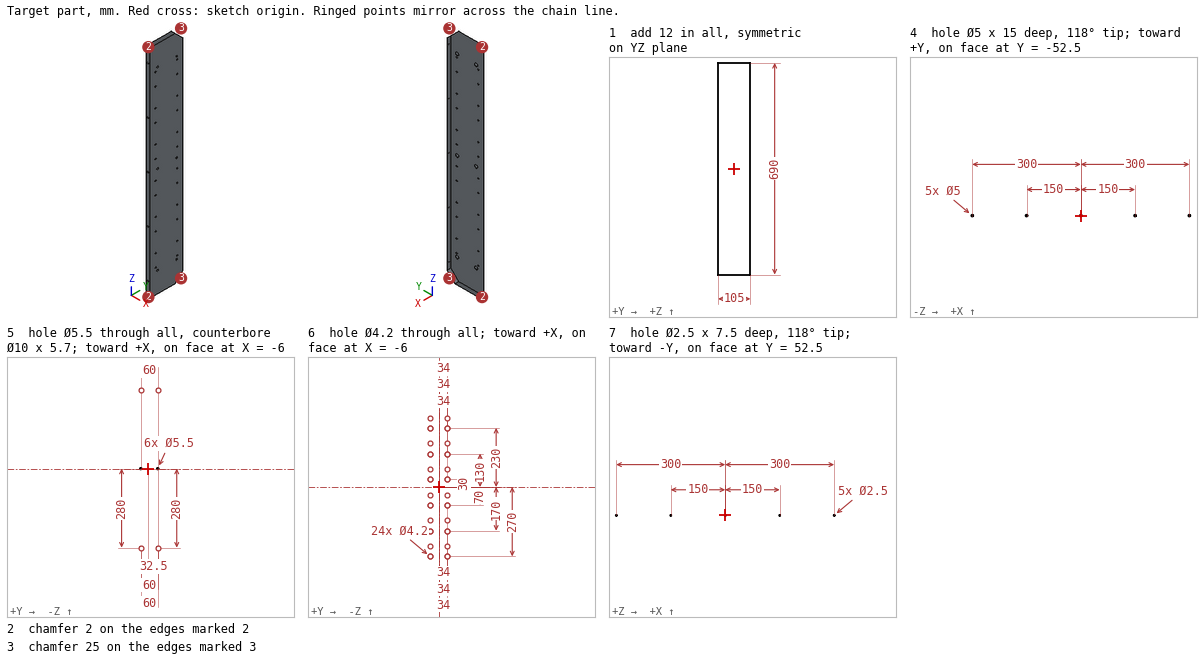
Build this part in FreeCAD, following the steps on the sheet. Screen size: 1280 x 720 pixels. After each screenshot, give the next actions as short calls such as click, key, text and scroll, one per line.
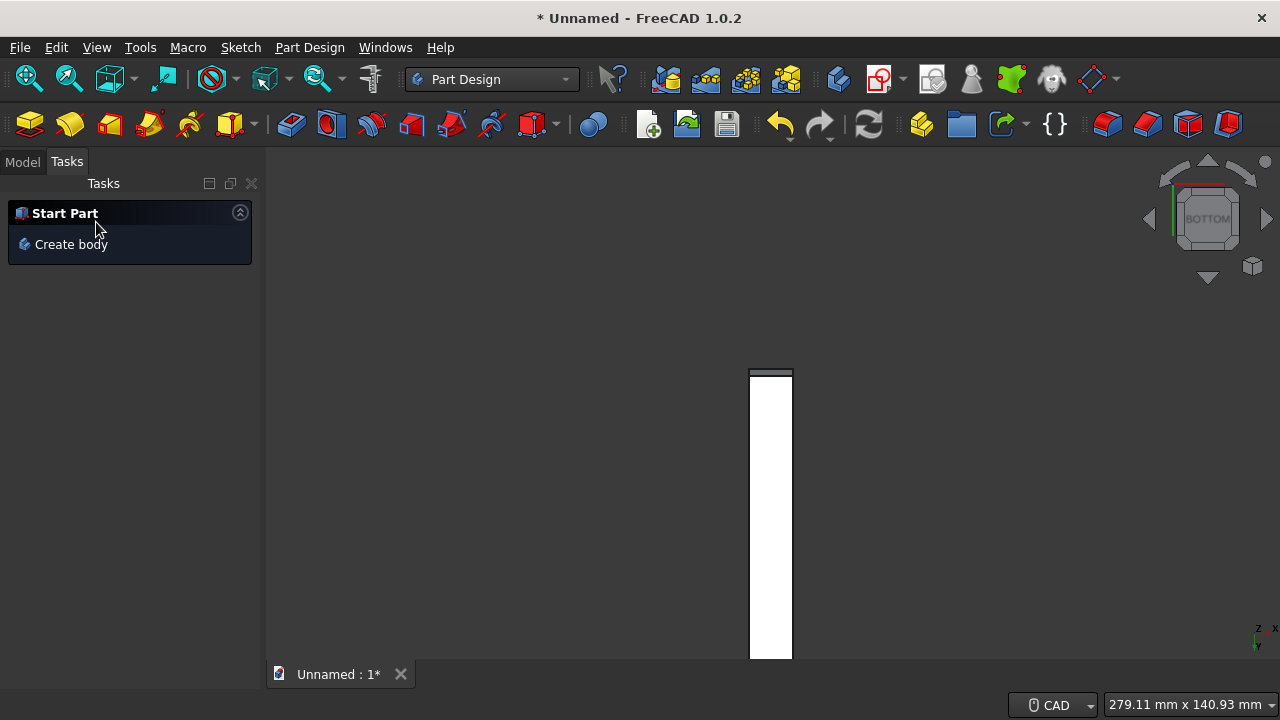
click(30, 80)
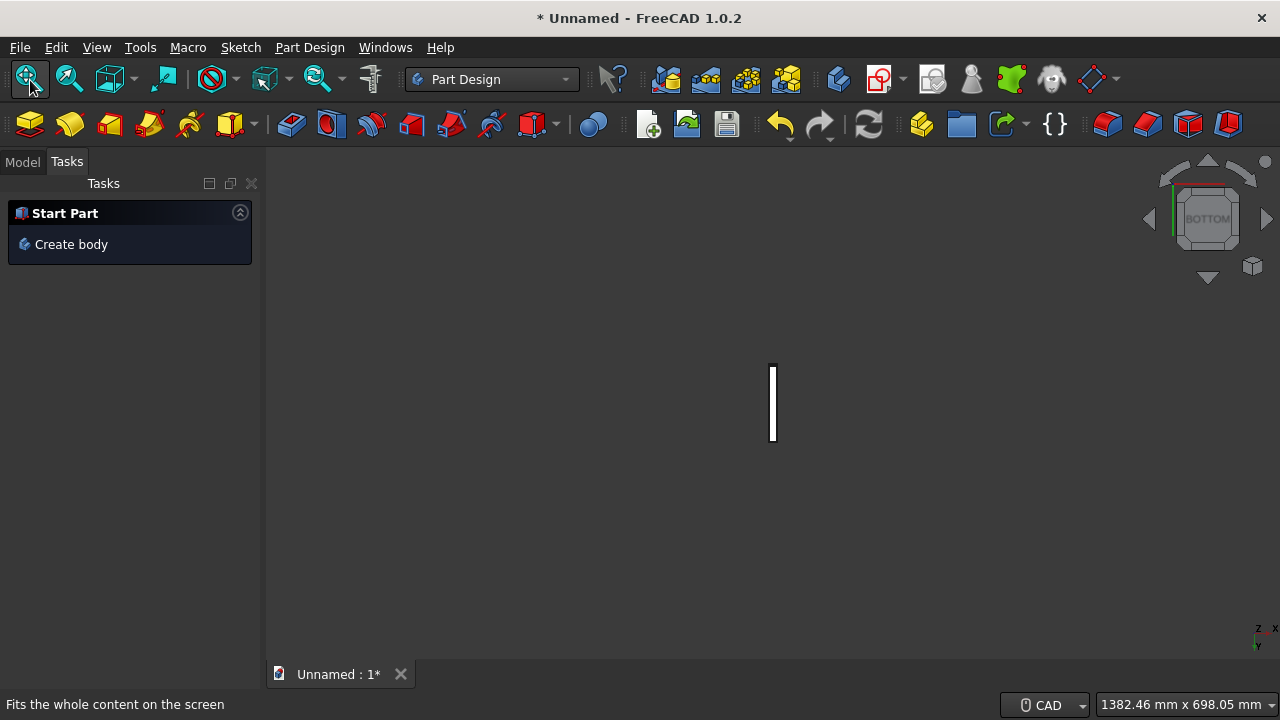
scroll(773, 441, up, 8)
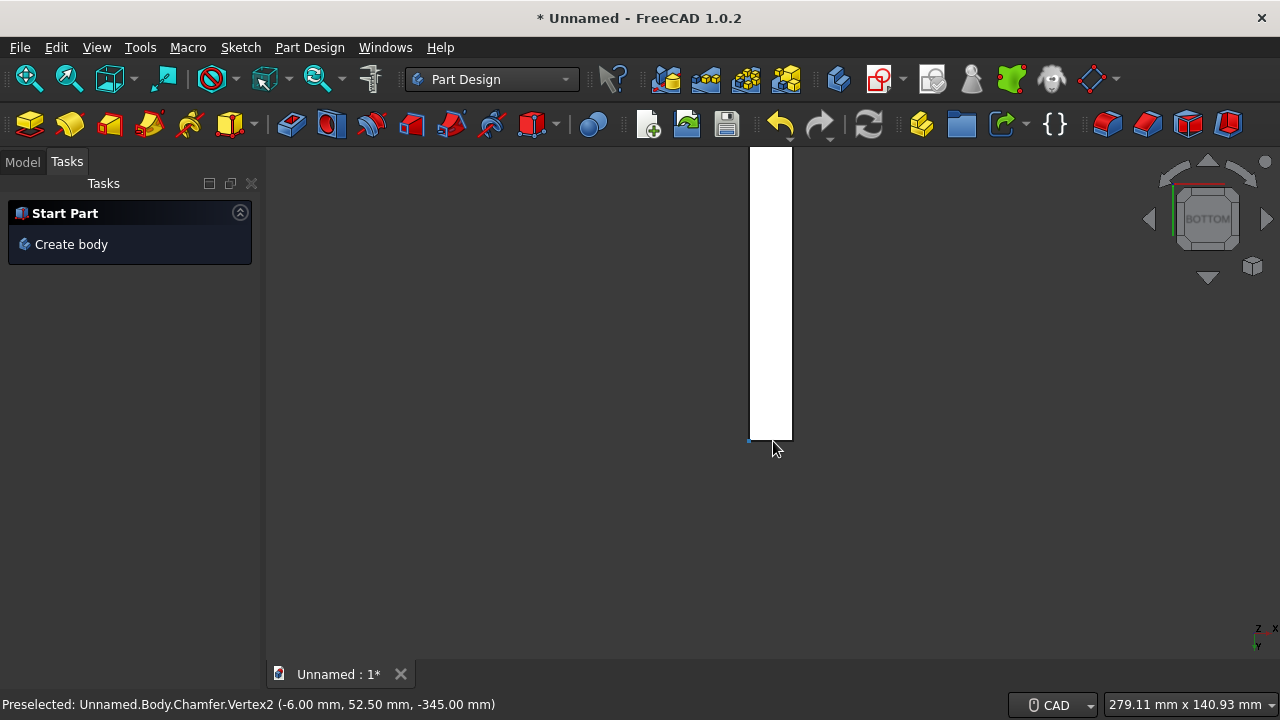
click(771, 440)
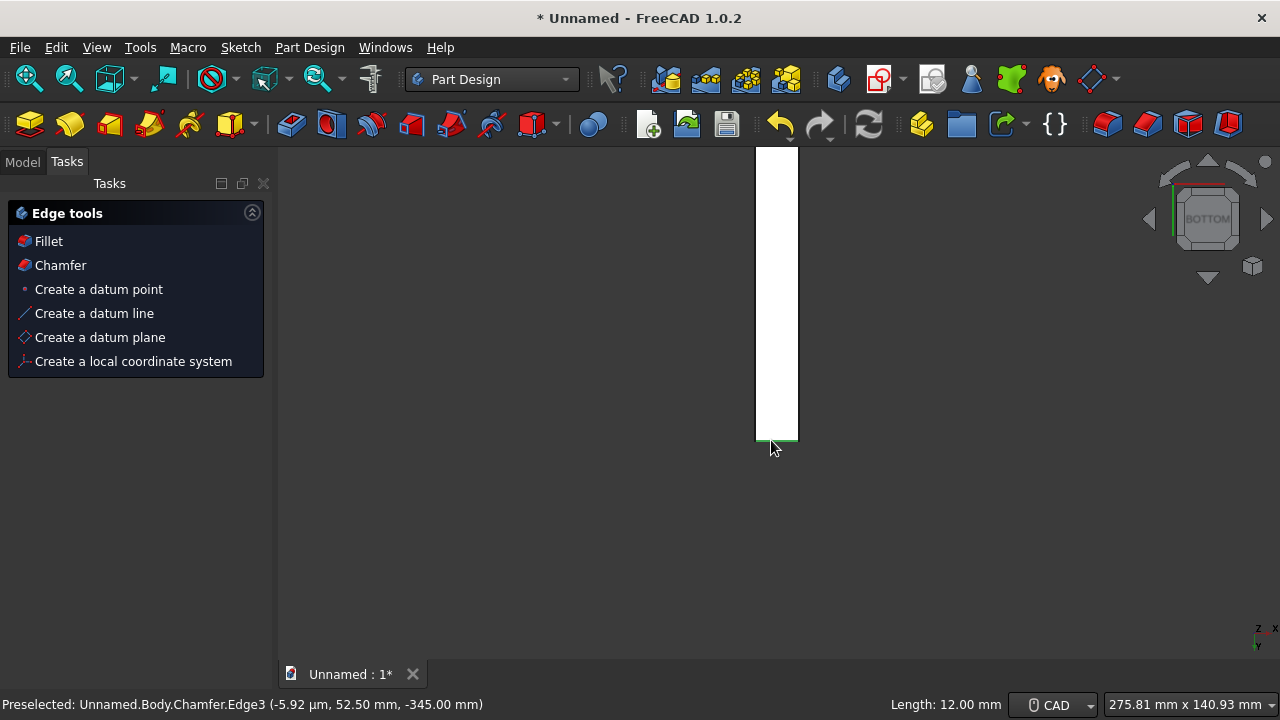
click(30, 80)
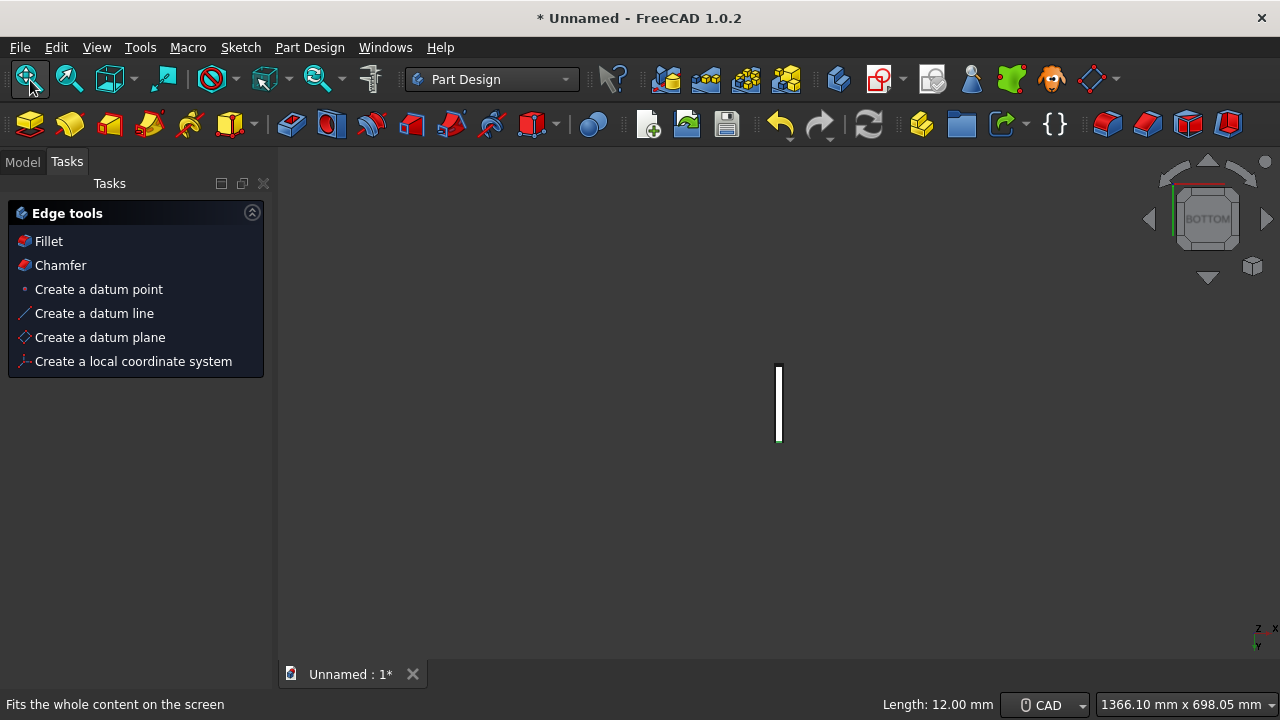
key(0)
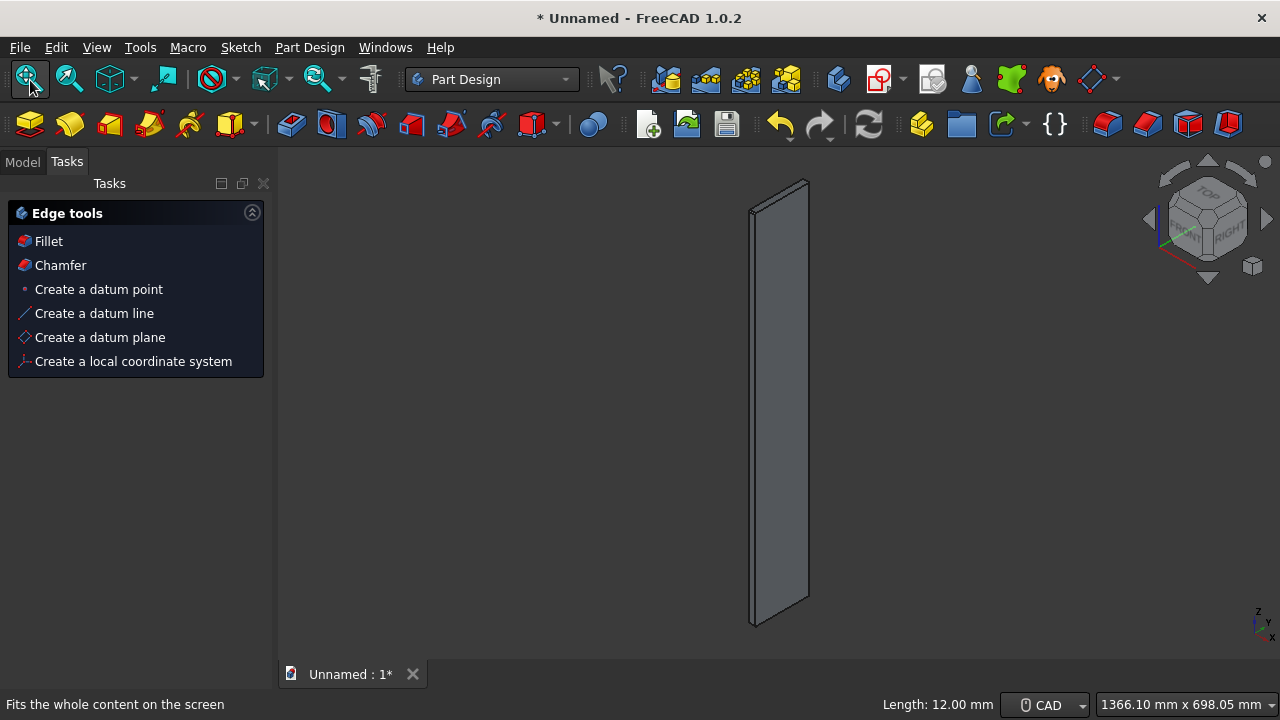
scroll(806, 180, up, 8)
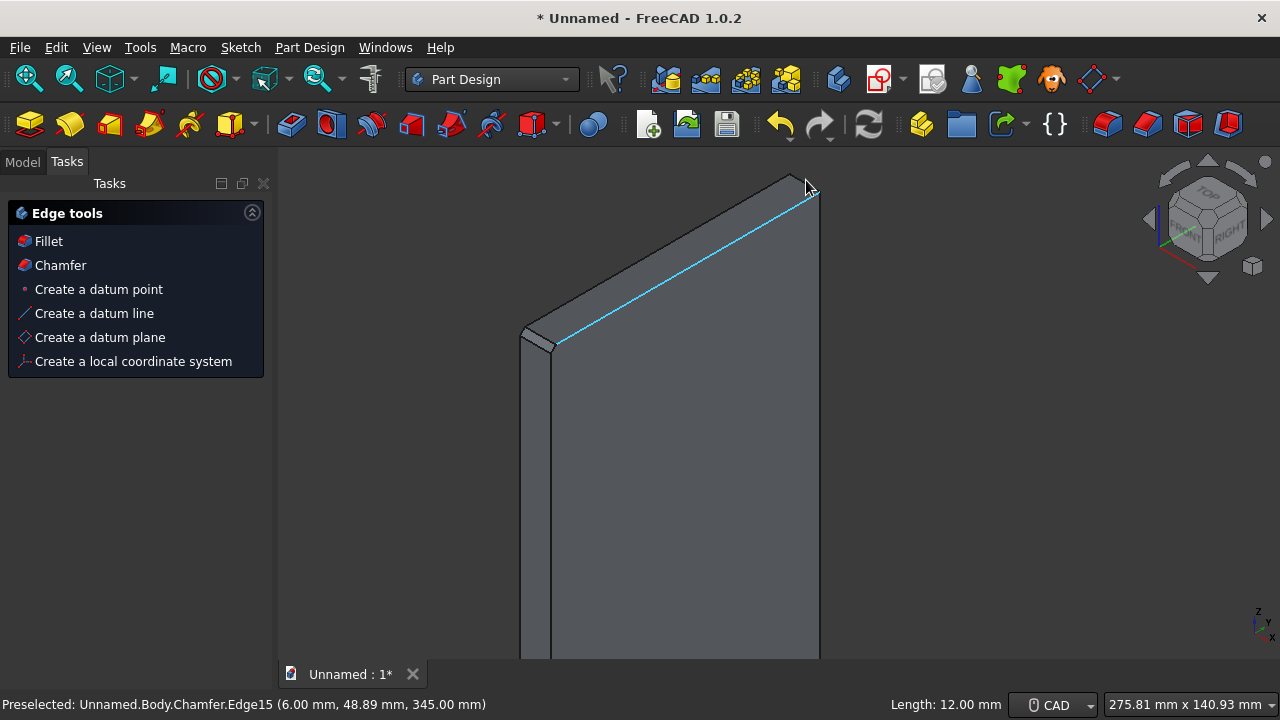
key(v)
key(f)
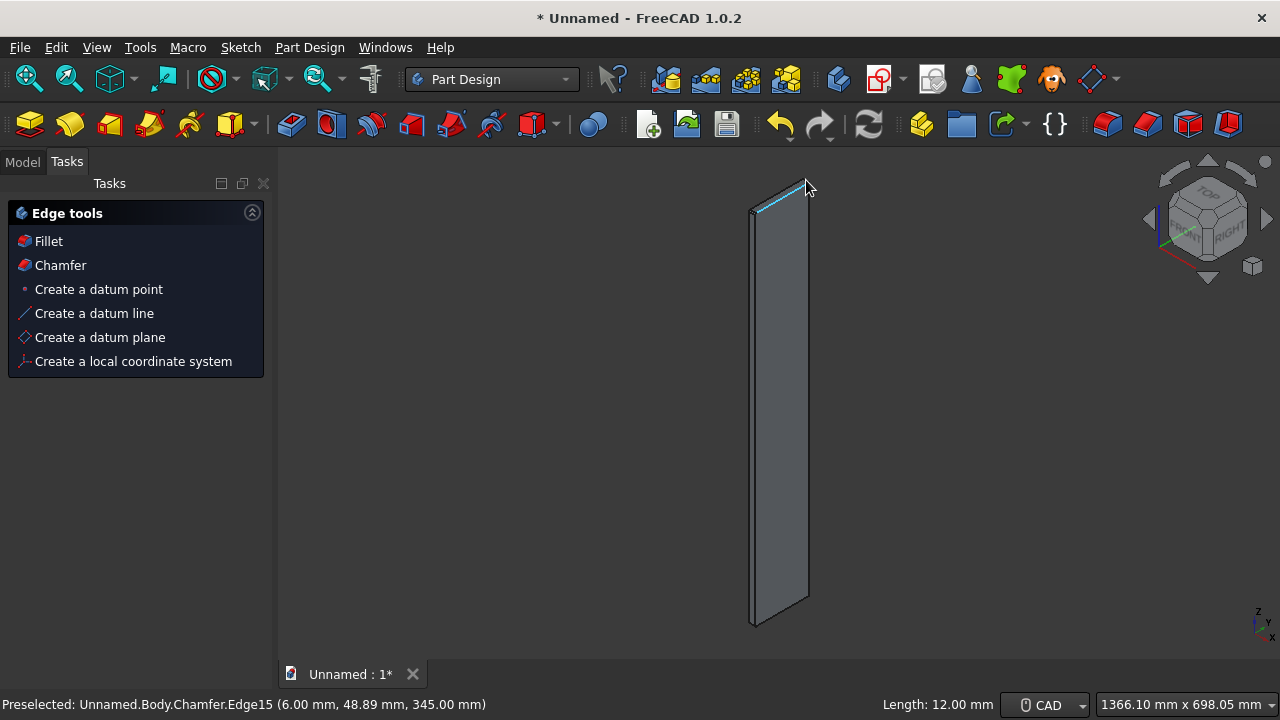
key(2)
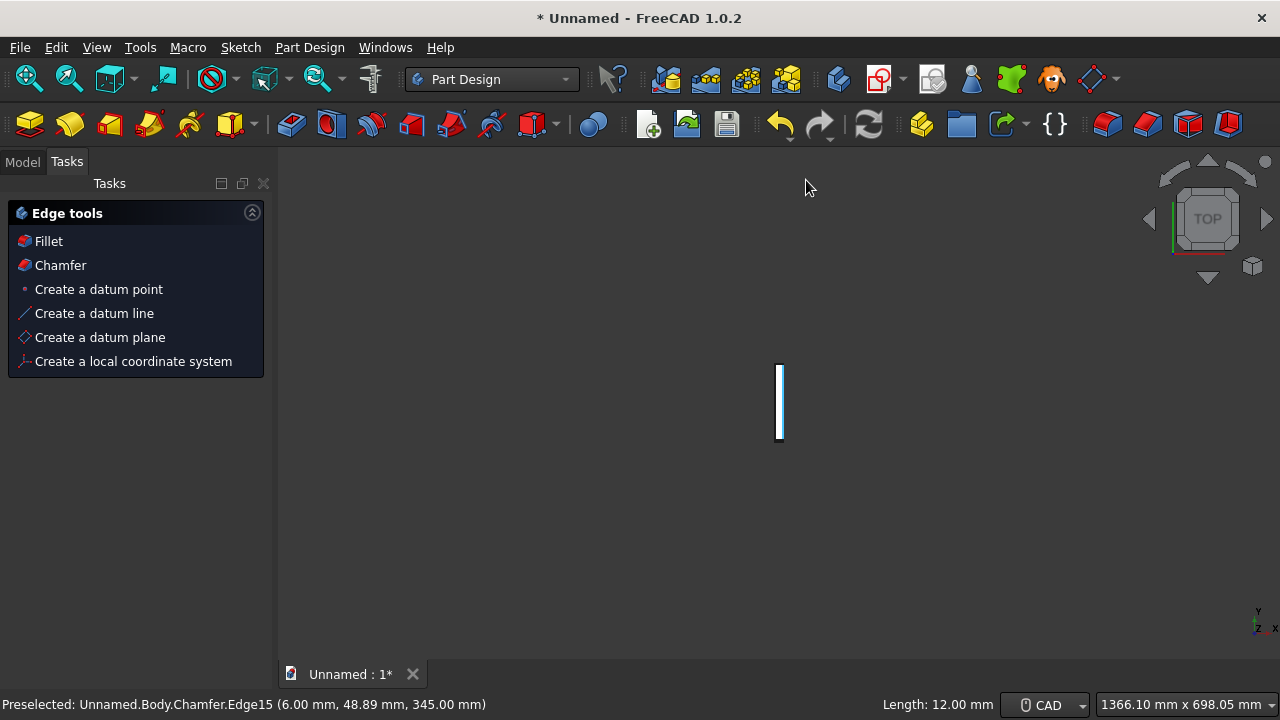
click(30, 80)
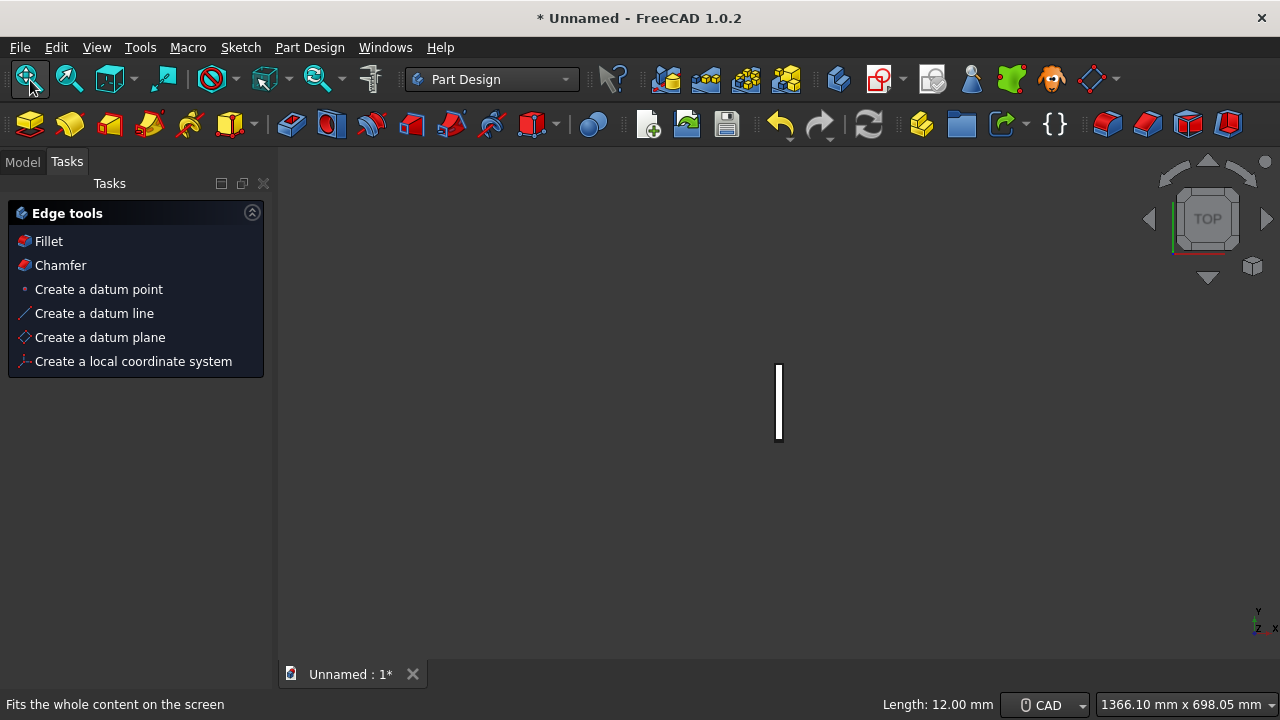
scroll(779, 363, up, 8)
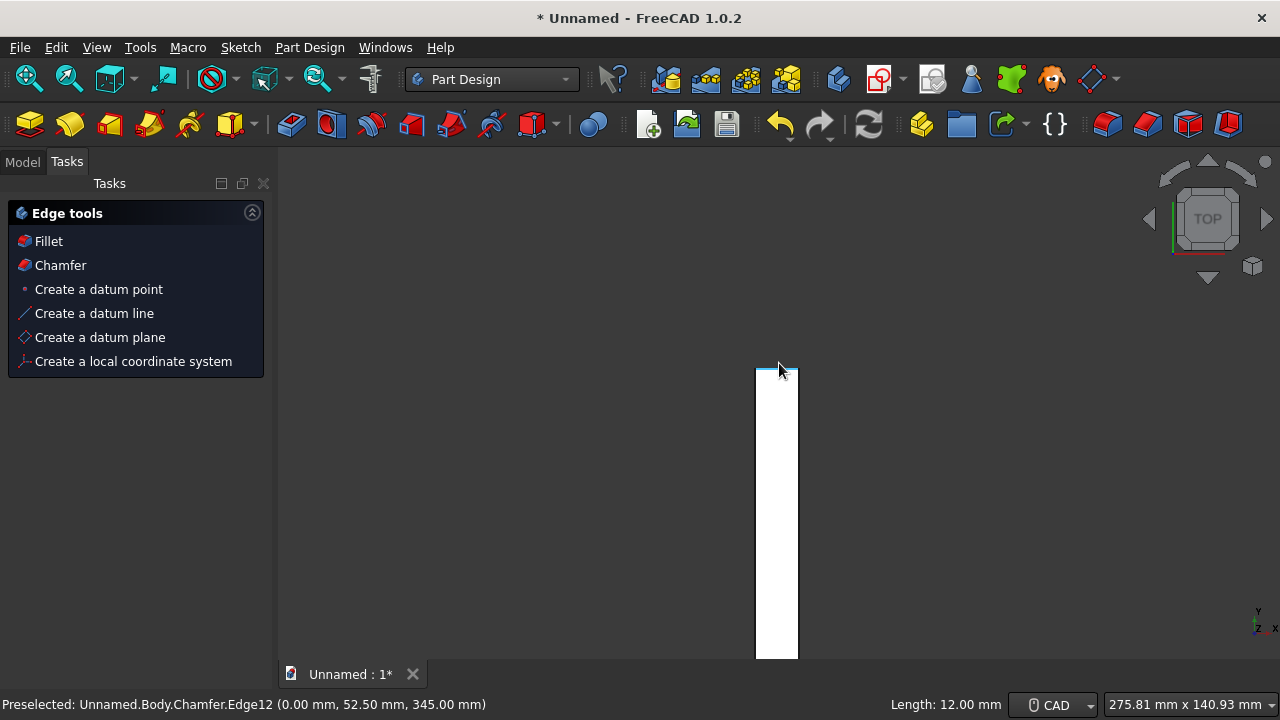
click(777, 368, ctrl)